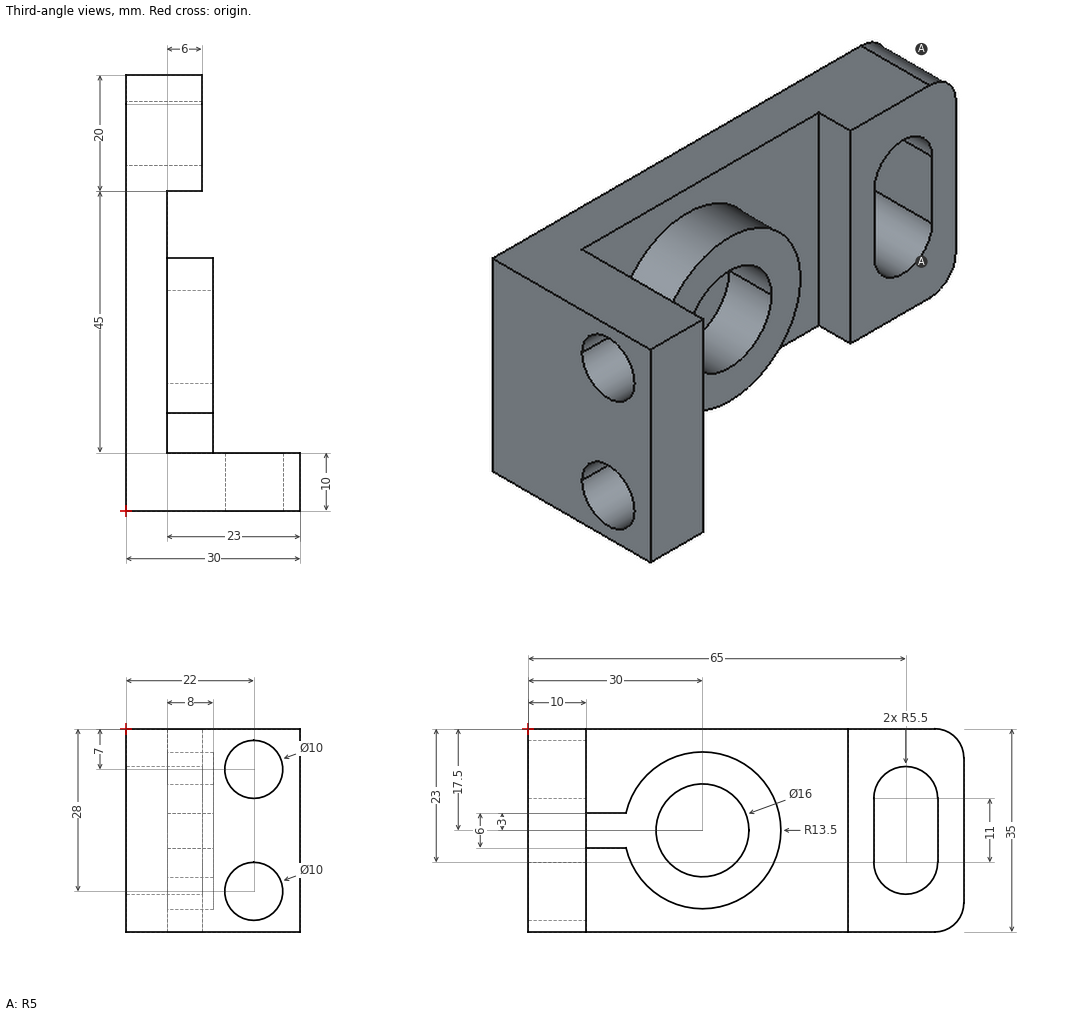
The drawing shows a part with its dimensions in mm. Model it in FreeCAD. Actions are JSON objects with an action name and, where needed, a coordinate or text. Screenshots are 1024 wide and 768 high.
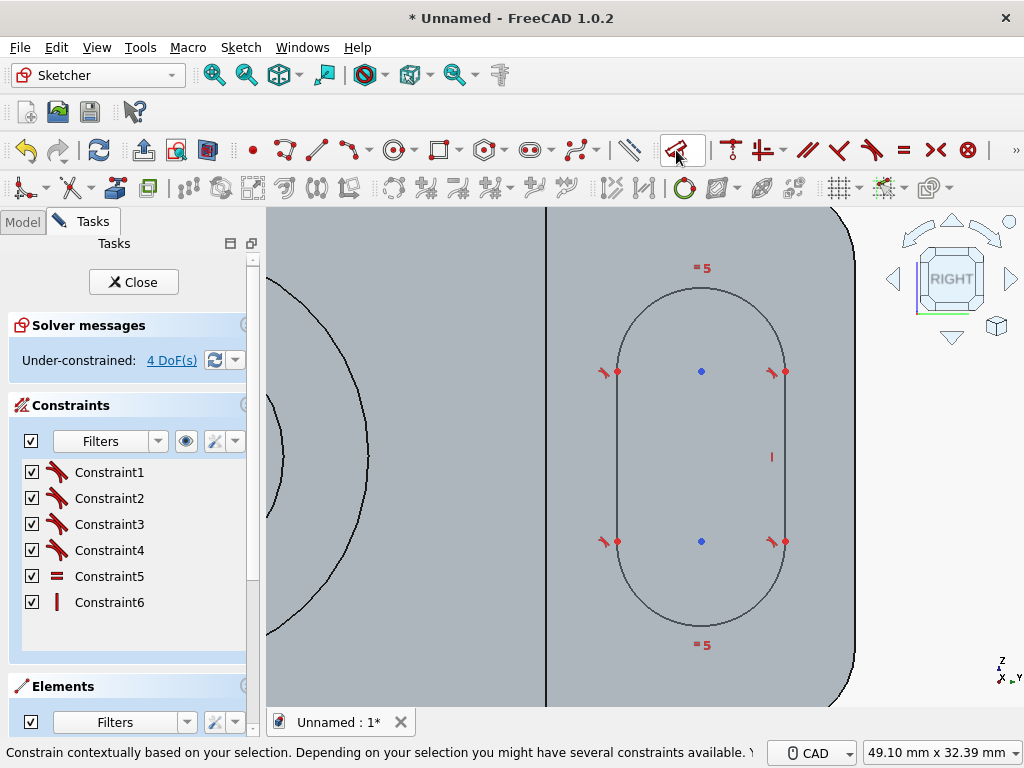
{"action": "left_click", "coordinate": [652, 610]}
{"action": "left_click", "coordinate": [633, 636]}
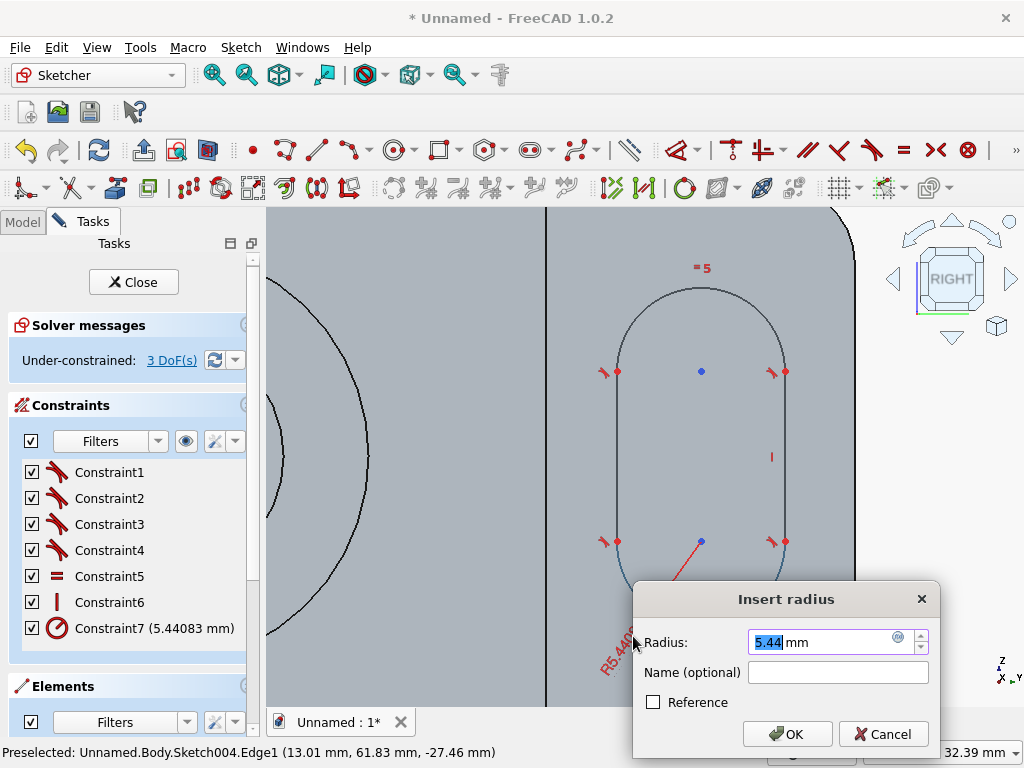
{"action": "type", "text": "5.5"}
{"action": "key", "text": "Return"}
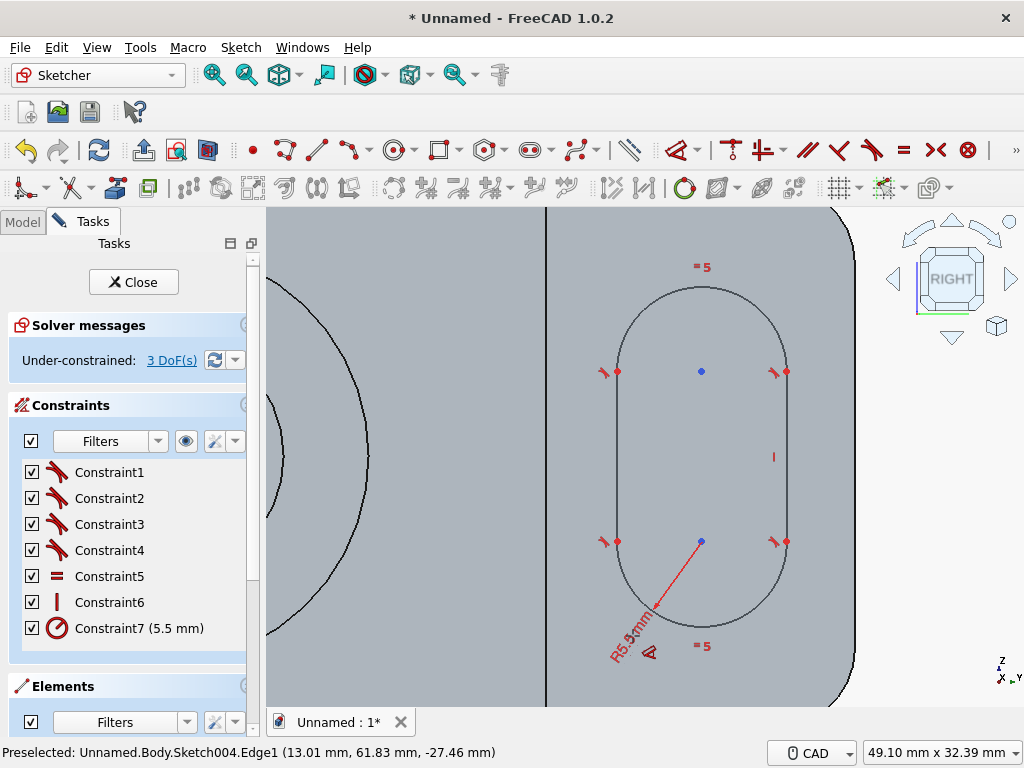
{"action": "left_click", "coordinate": [617, 491]}
{"action": "left_click", "coordinate": [583, 457]}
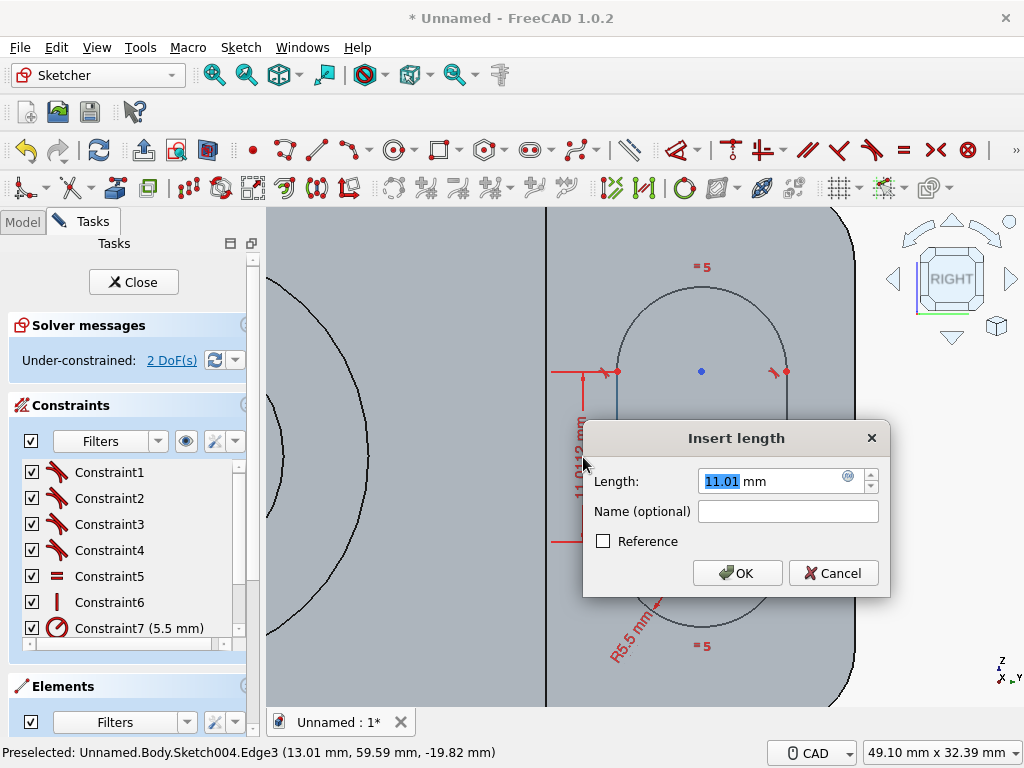
{"action": "type", "text": "11"}
{"action": "key", "text": "Return"}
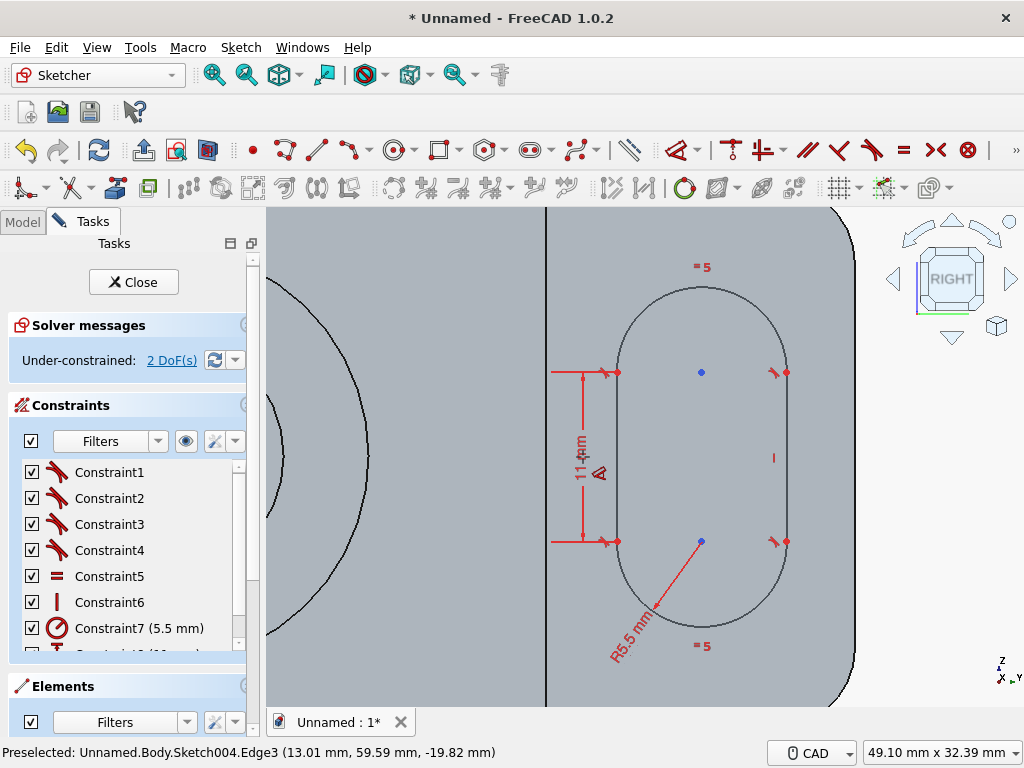
{"action": "left_click", "coordinate": [617, 542]}
{"action": "left_click", "coordinate": [651, 388]}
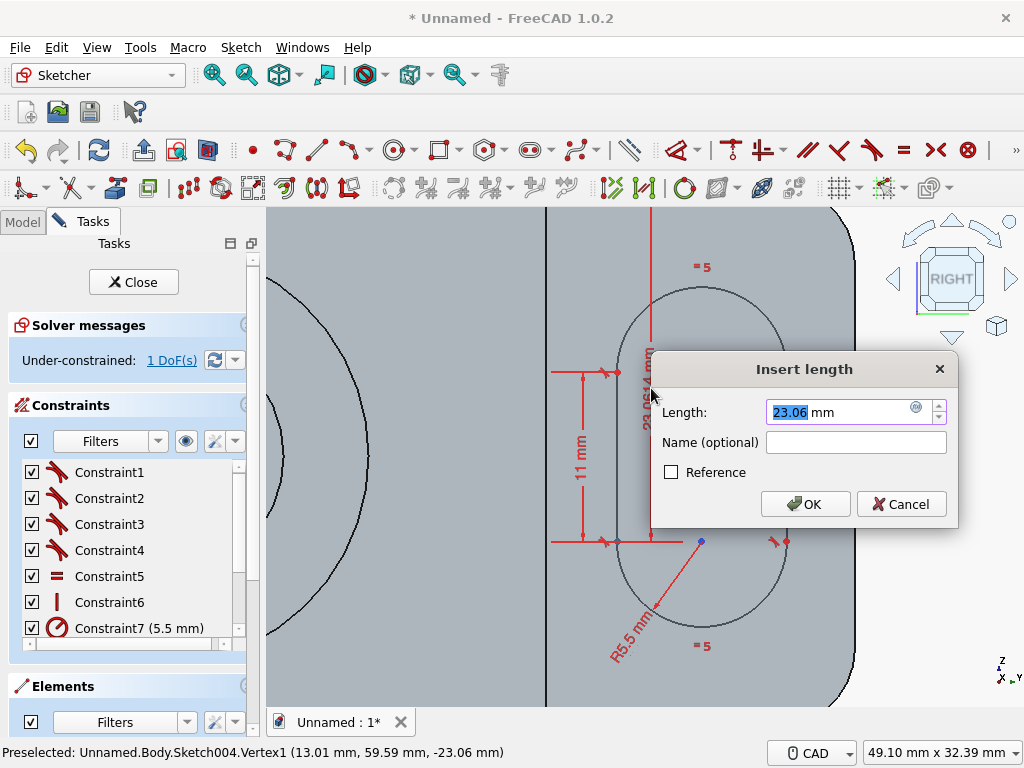
{"action": "type", "text": "23"}
{"action": "key", "text": "Return"}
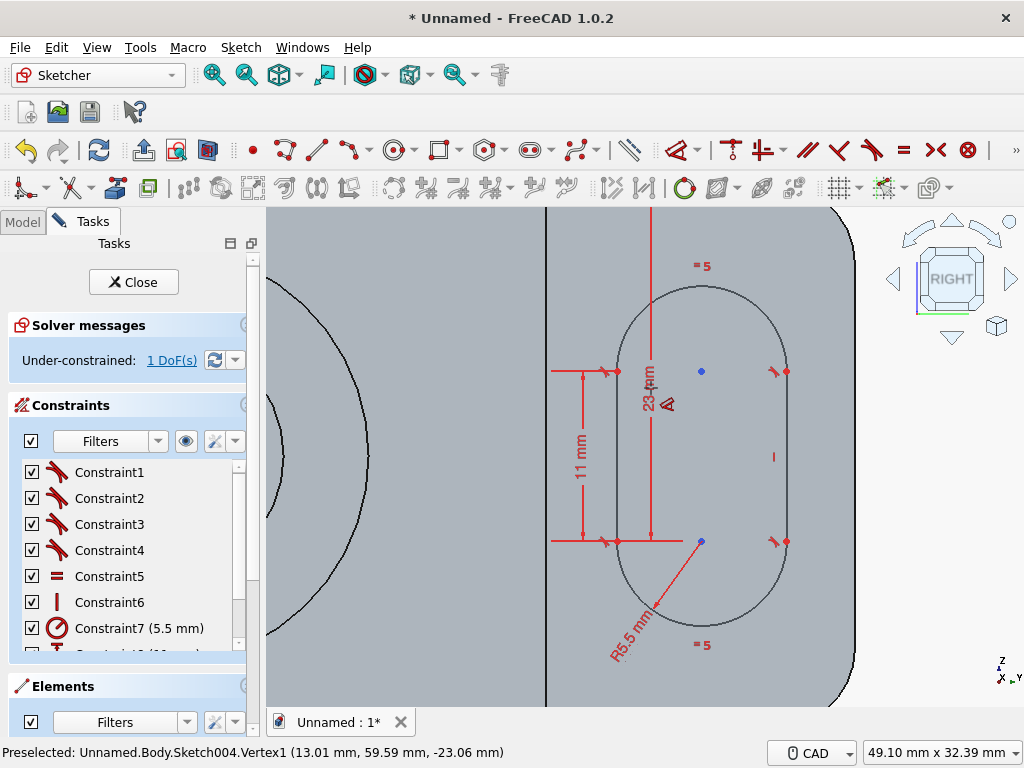
{"action": "left_click", "coordinate": [702, 541]}
{"action": "left_click", "coordinate": [498, 575]}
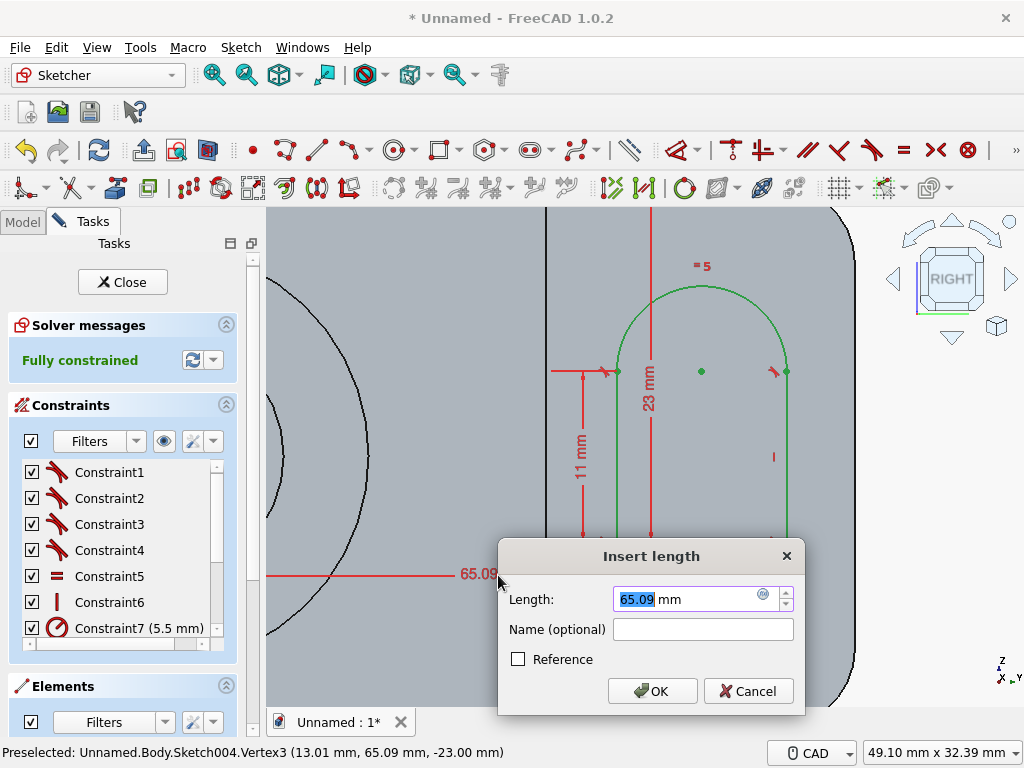
{"action": "type", "text": "65"}
{"action": "key", "text": "Return"}
{"action": "key", "text": "Escape"}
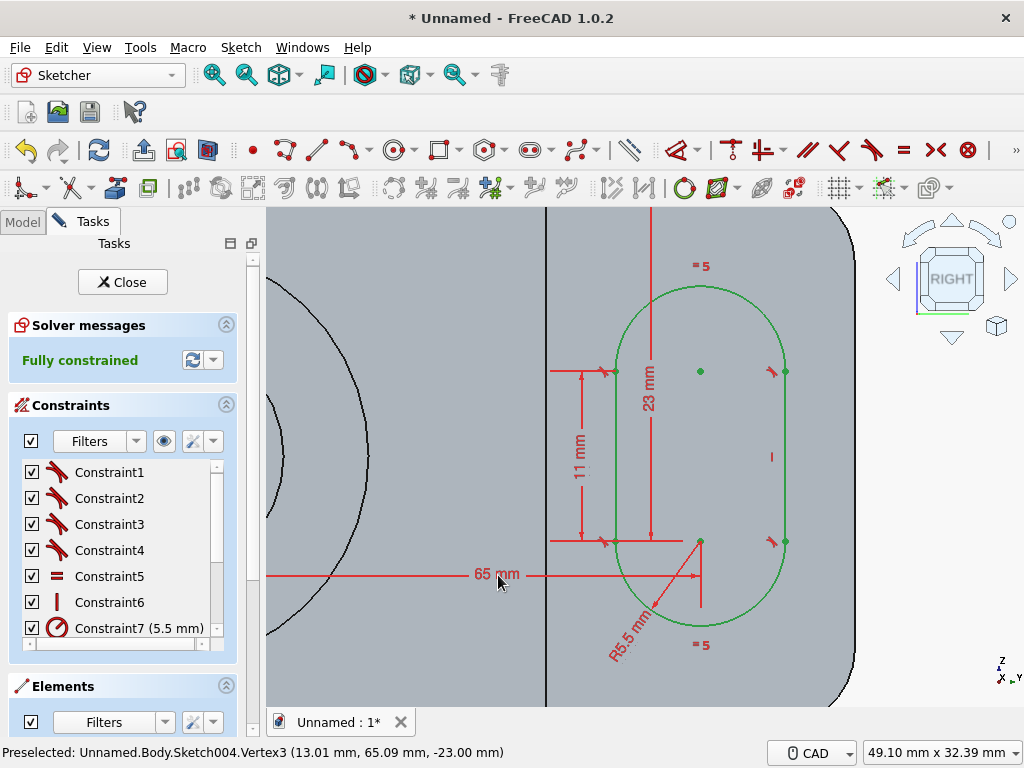
{"action": "left_click", "coordinate": [123, 282]}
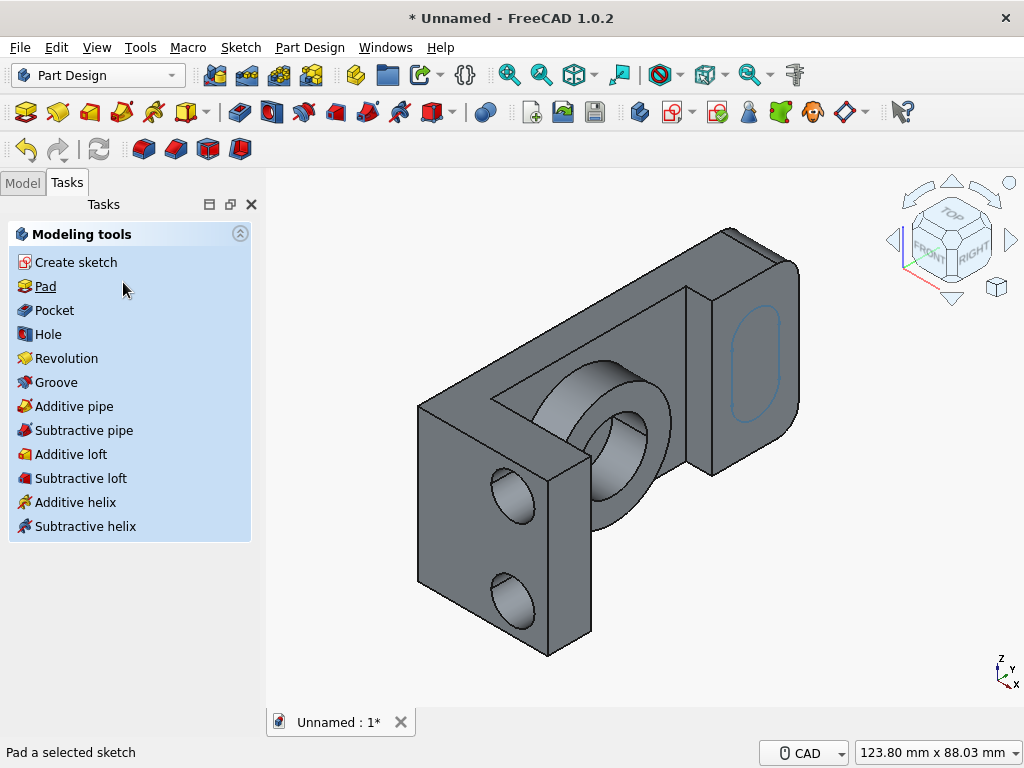
{"action": "left_click", "coordinate": [240, 112]}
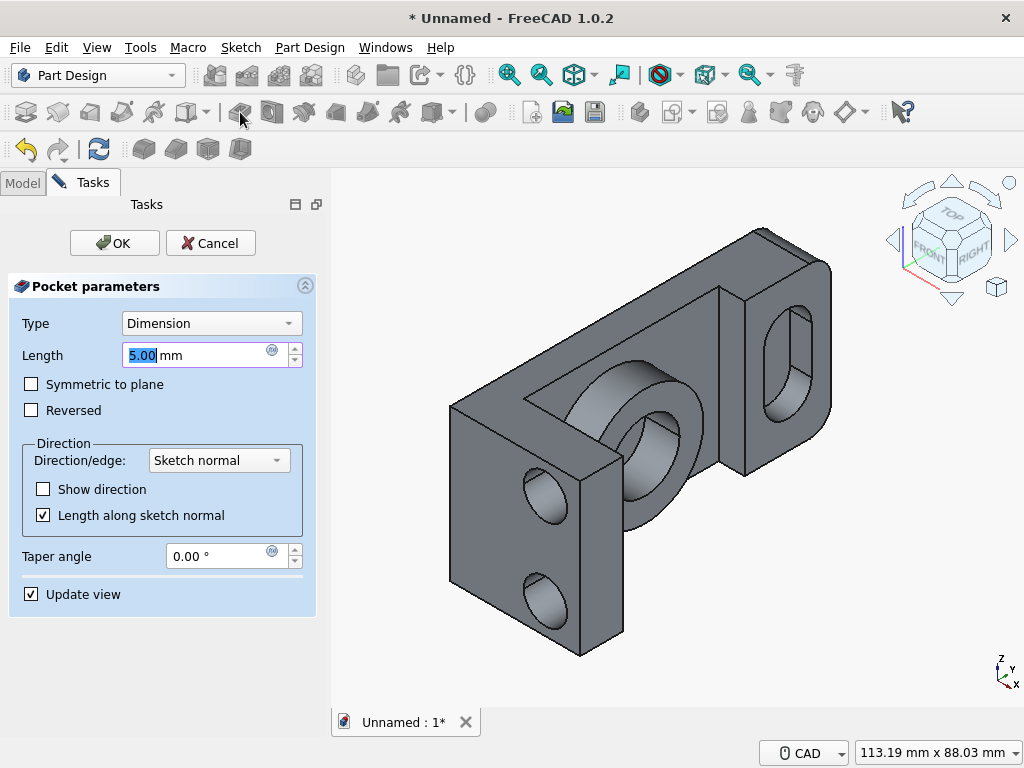
{"action": "left_click", "coordinate": [212, 324]}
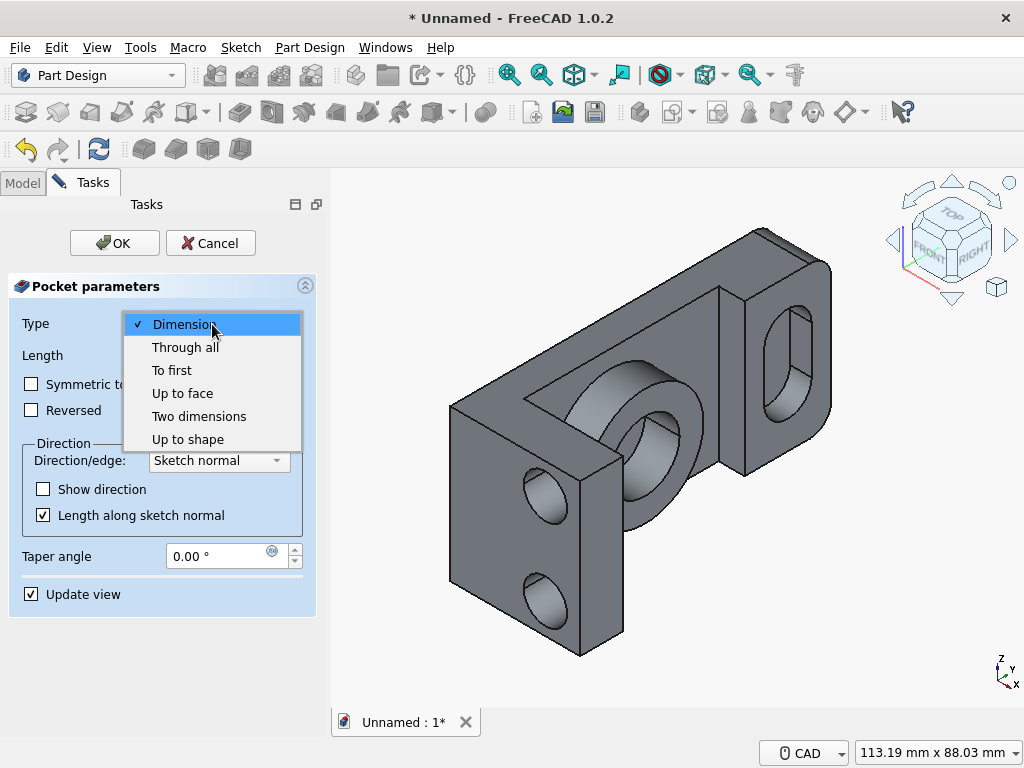
{"action": "left_click", "coordinate": [212, 370]}